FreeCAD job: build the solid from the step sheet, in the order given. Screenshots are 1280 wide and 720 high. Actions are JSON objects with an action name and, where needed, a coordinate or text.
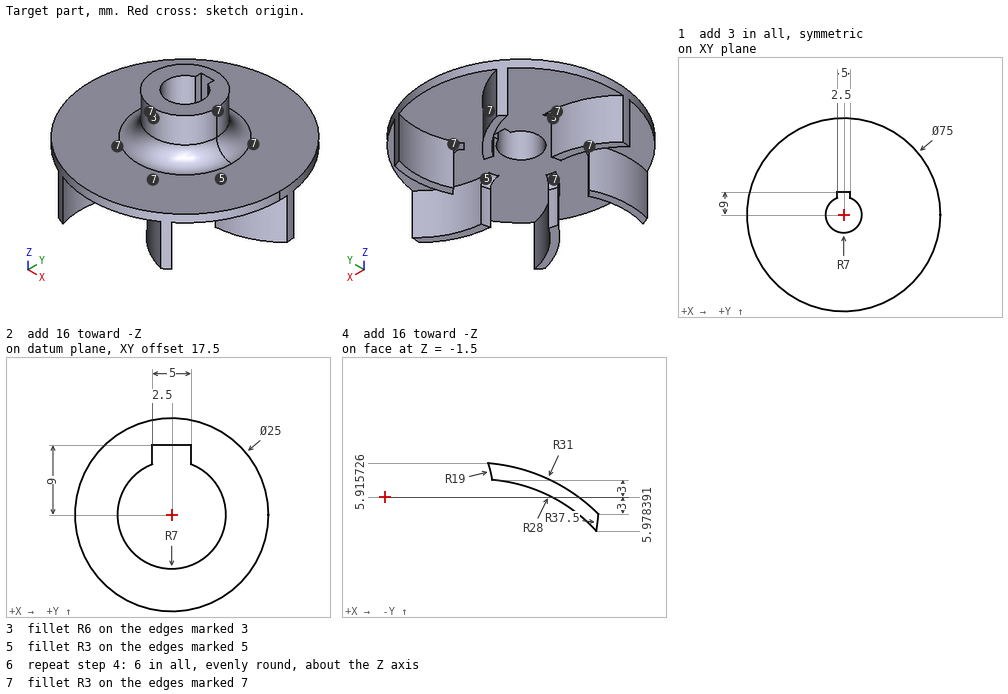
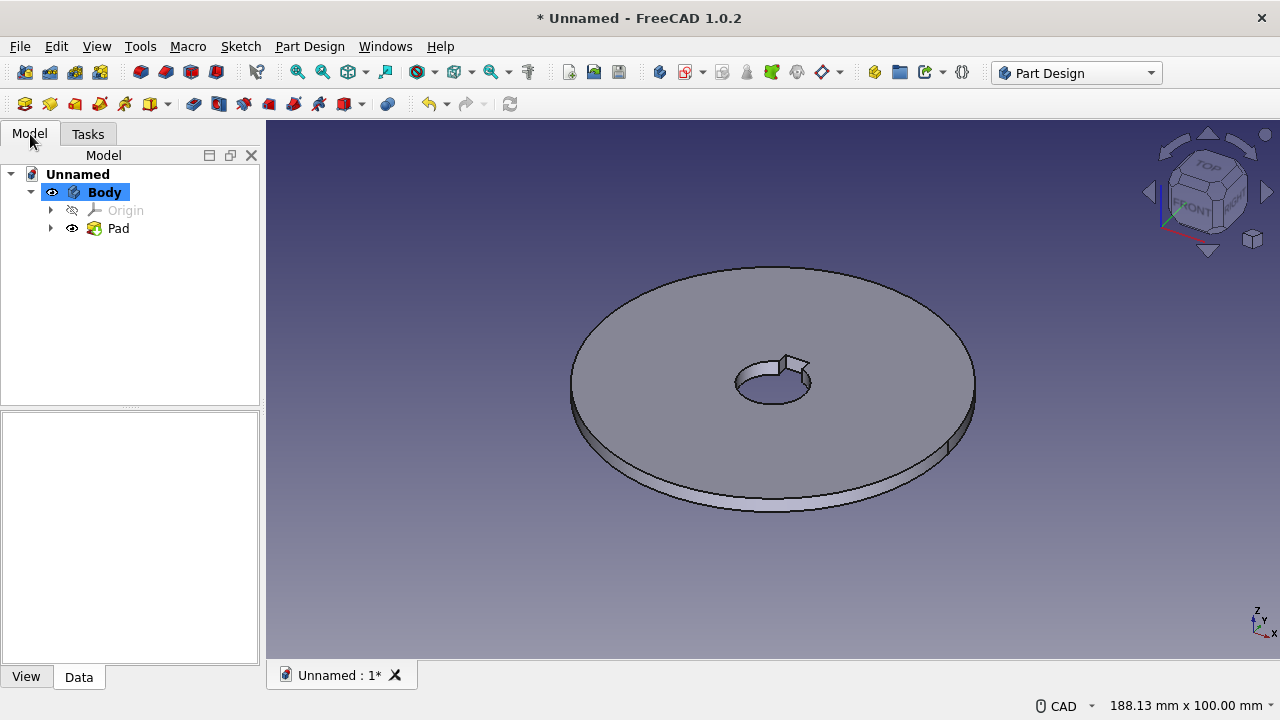
{"action": "left_click", "coordinate": [51, 210]}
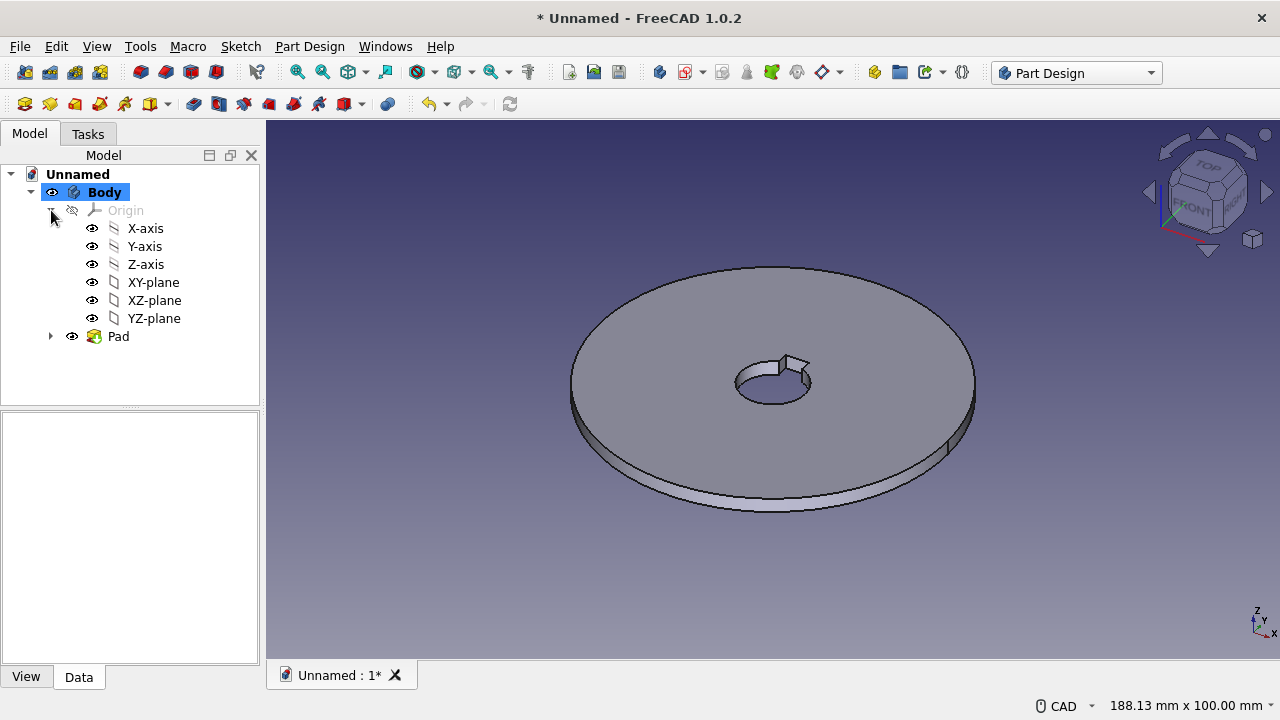
{"action": "left_click", "coordinate": [137, 282]}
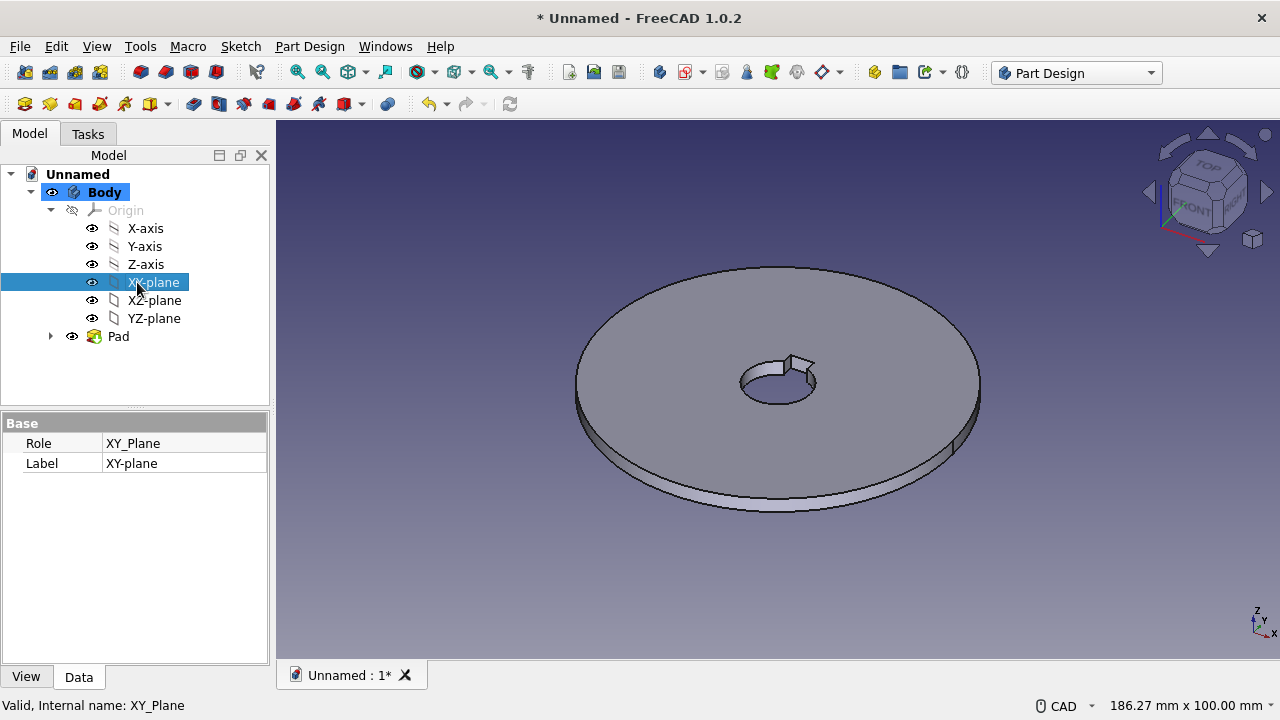
{"action": "left_click", "coordinate": [822, 72]}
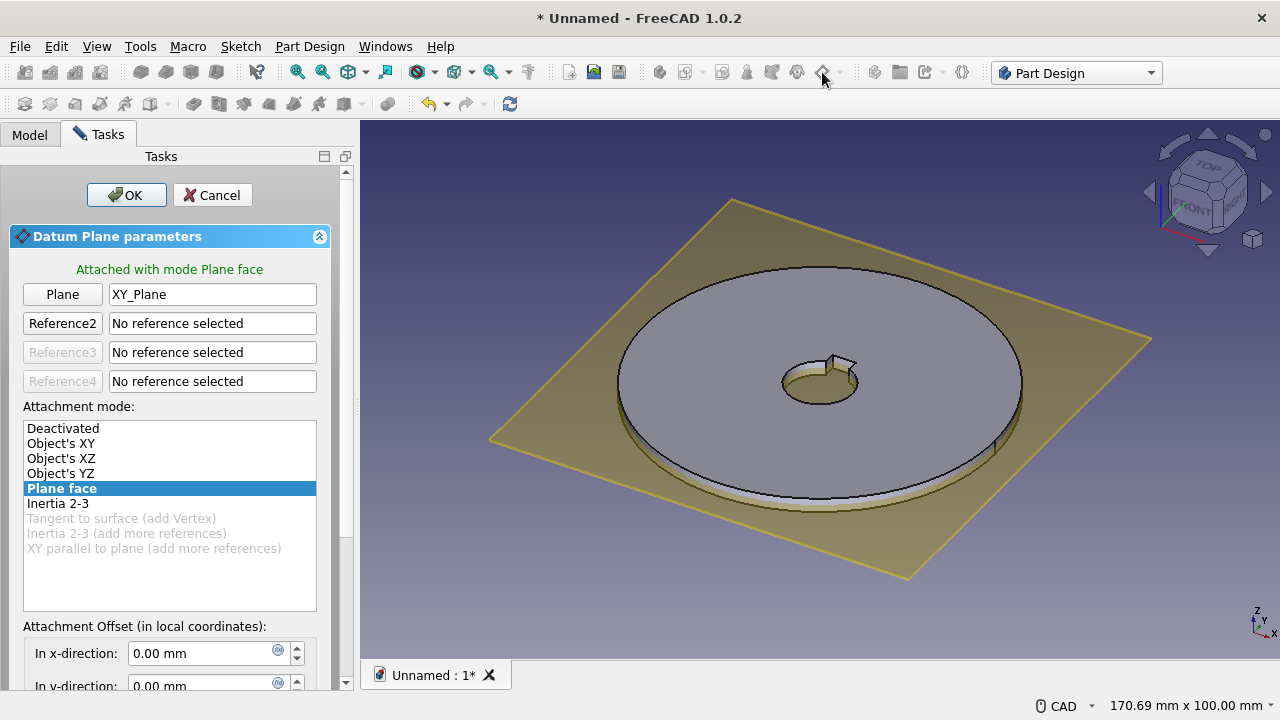
{"action": "scroll", "coordinate": [346, 428], "scroll_direction": "down", "scroll_amount": 2}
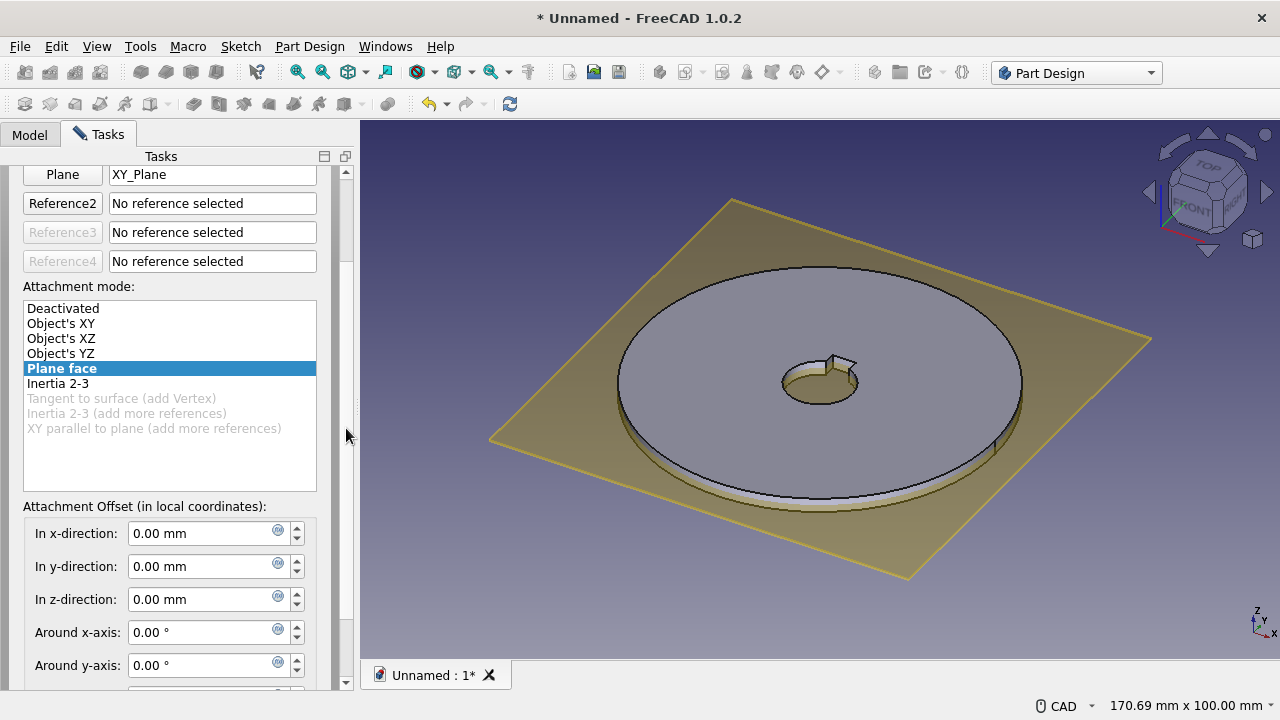
{"action": "triple_click", "coordinate": [210, 600]}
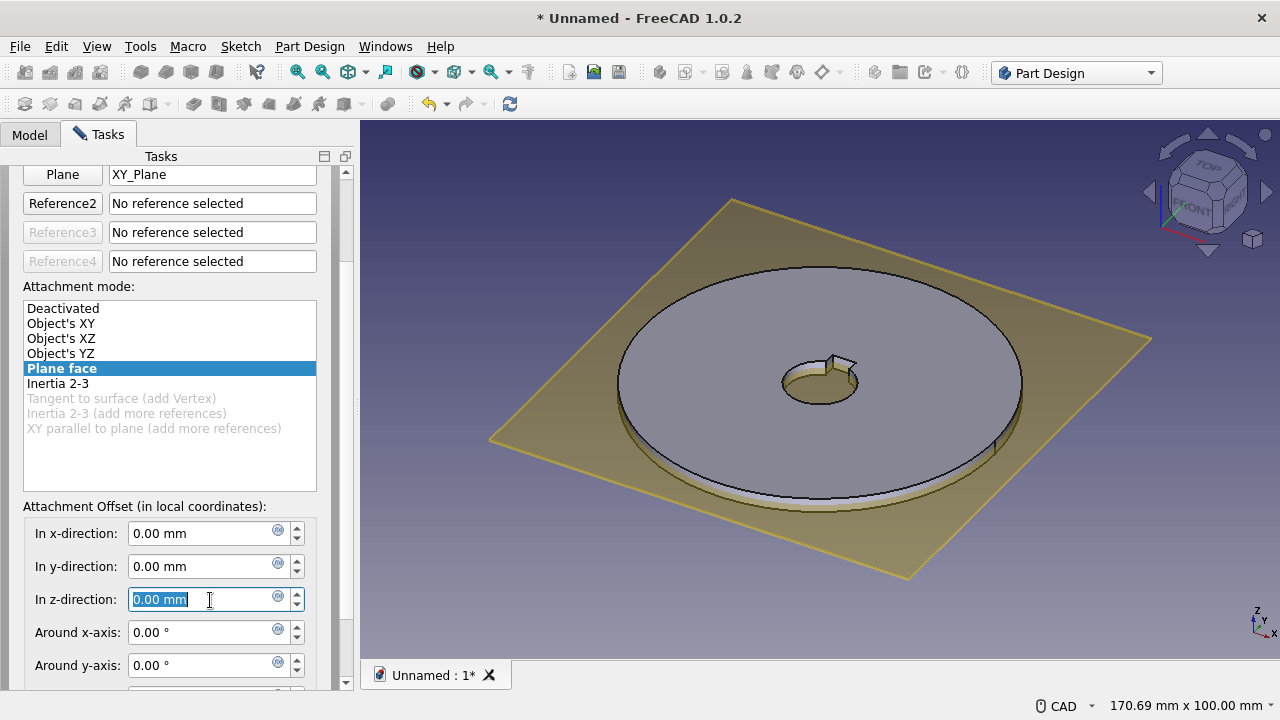
{"action": "type", "text": "17.5"}
{"action": "key", "text": "Tab"}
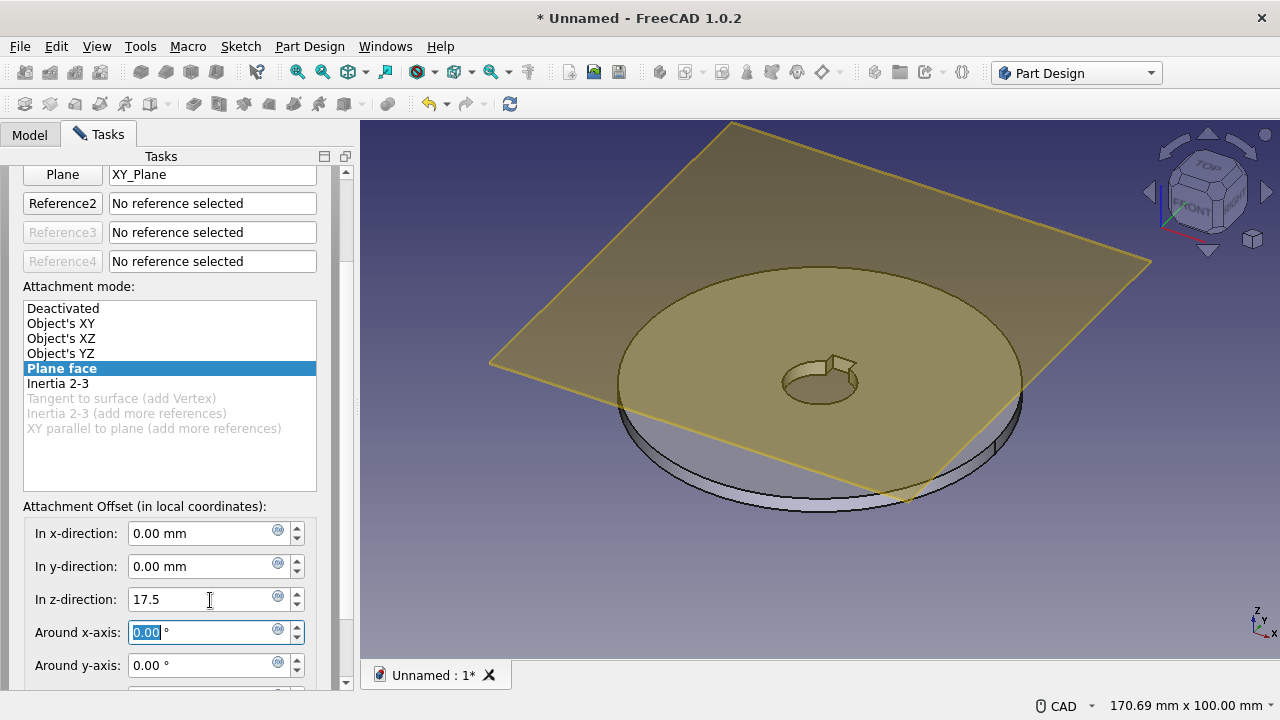
{"action": "scroll", "coordinate": [346, 428], "scroll_direction": "up", "scroll_amount": 3}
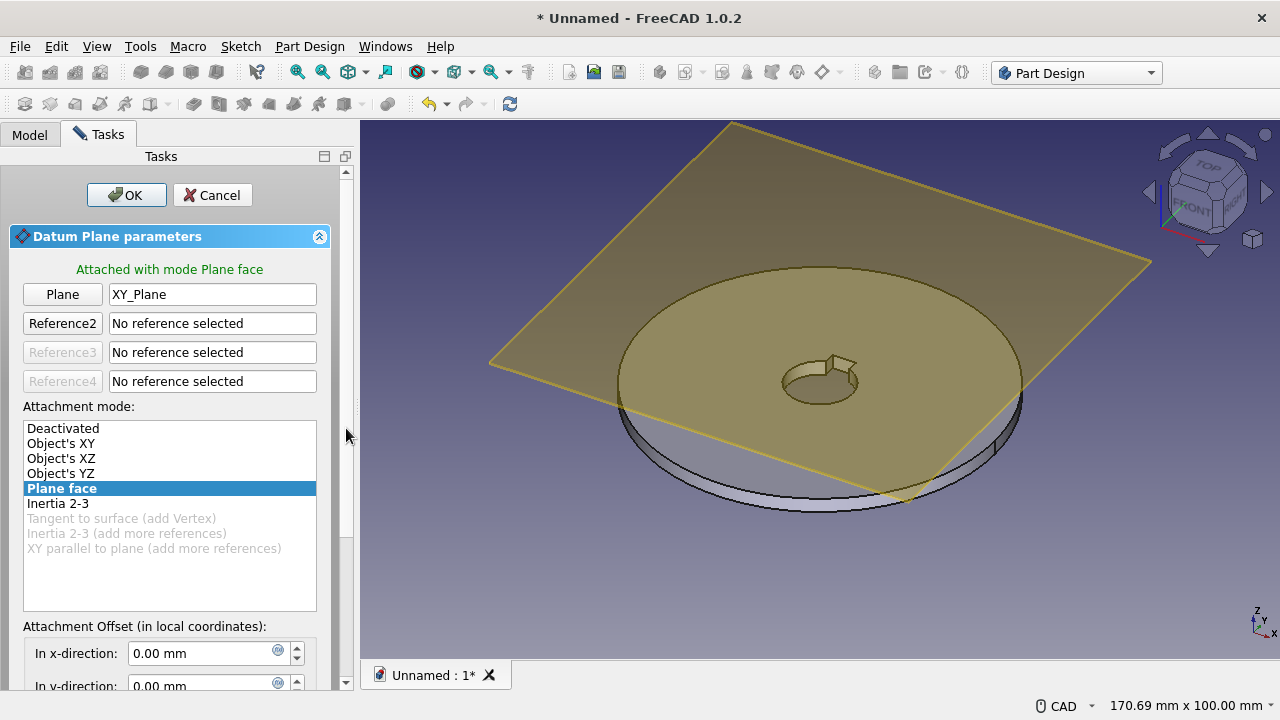
{"action": "left_click", "coordinate": [127, 195]}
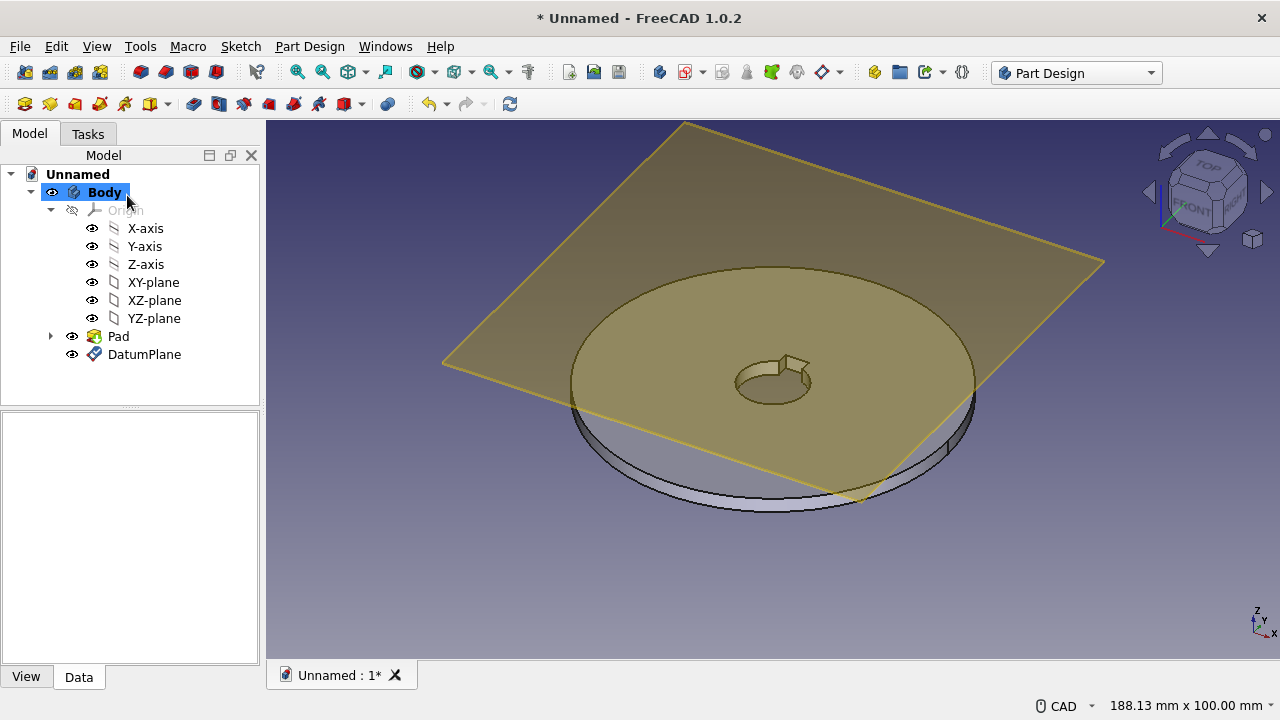
{"action": "left_click", "coordinate": [117, 354]}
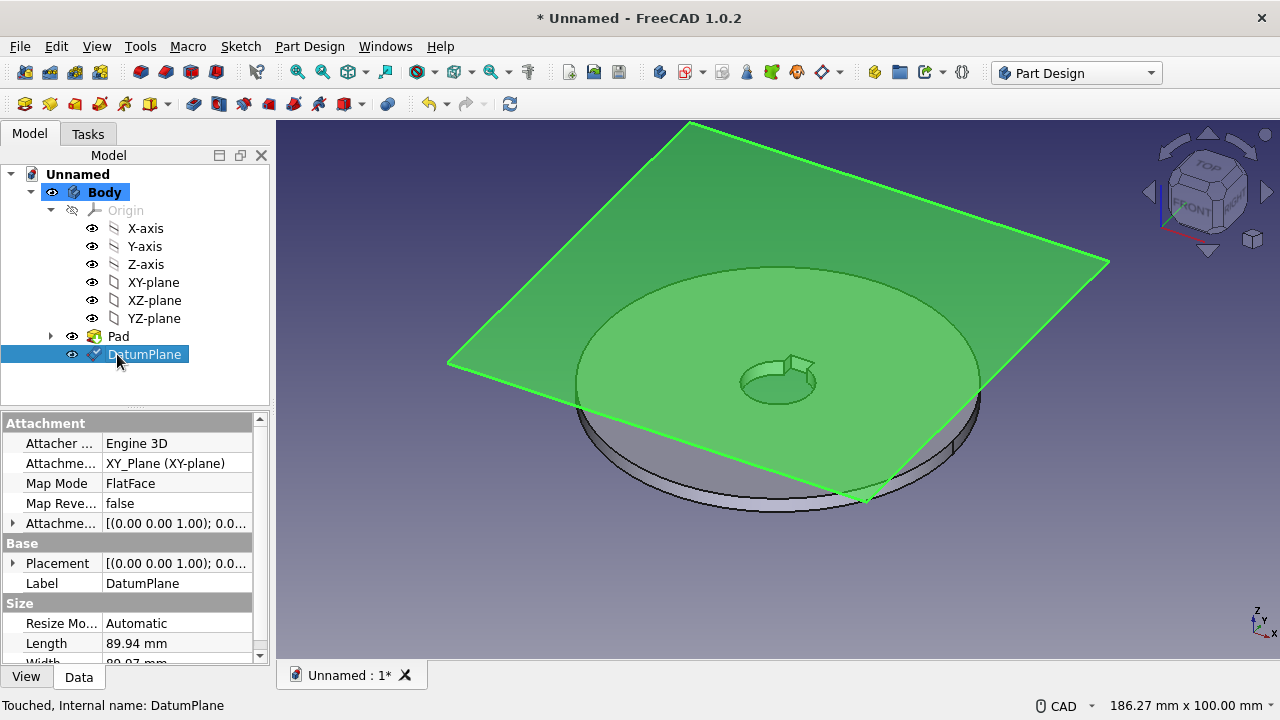
{"action": "left_click", "coordinate": [684, 72]}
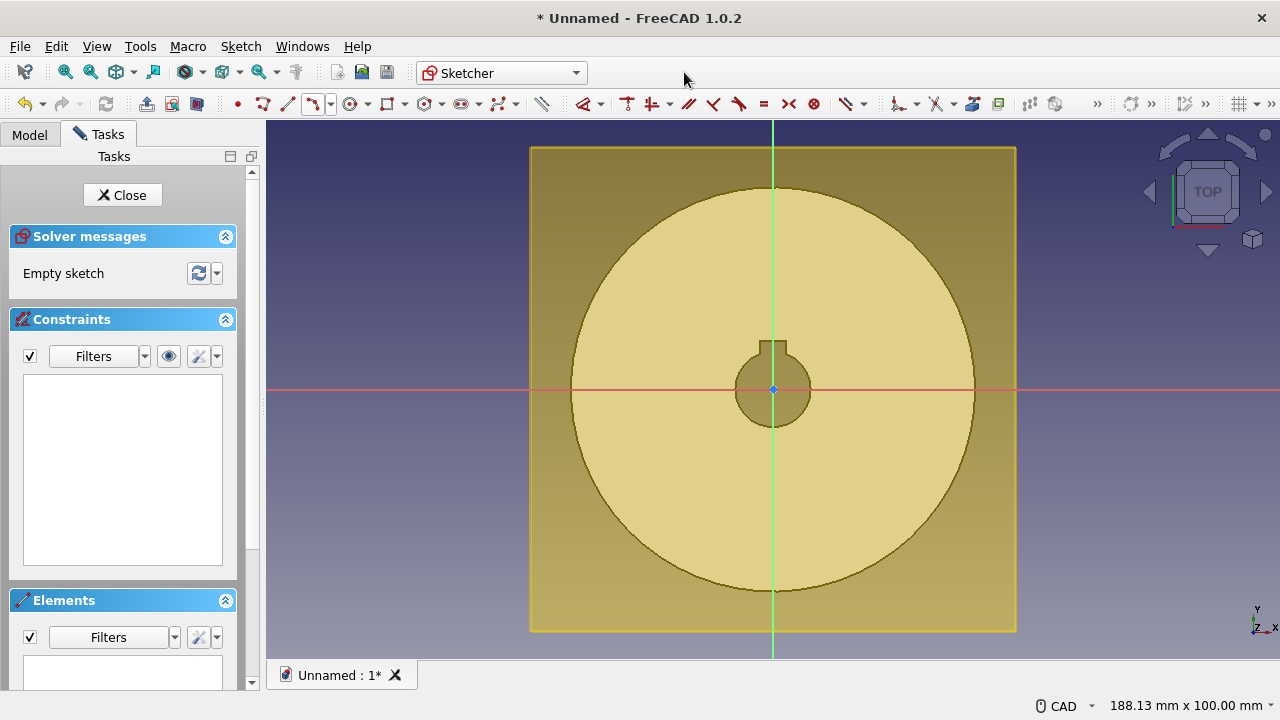
{"action": "scroll", "coordinate": [813, 390], "scroll_direction": "up", "scroll_amount": 5}